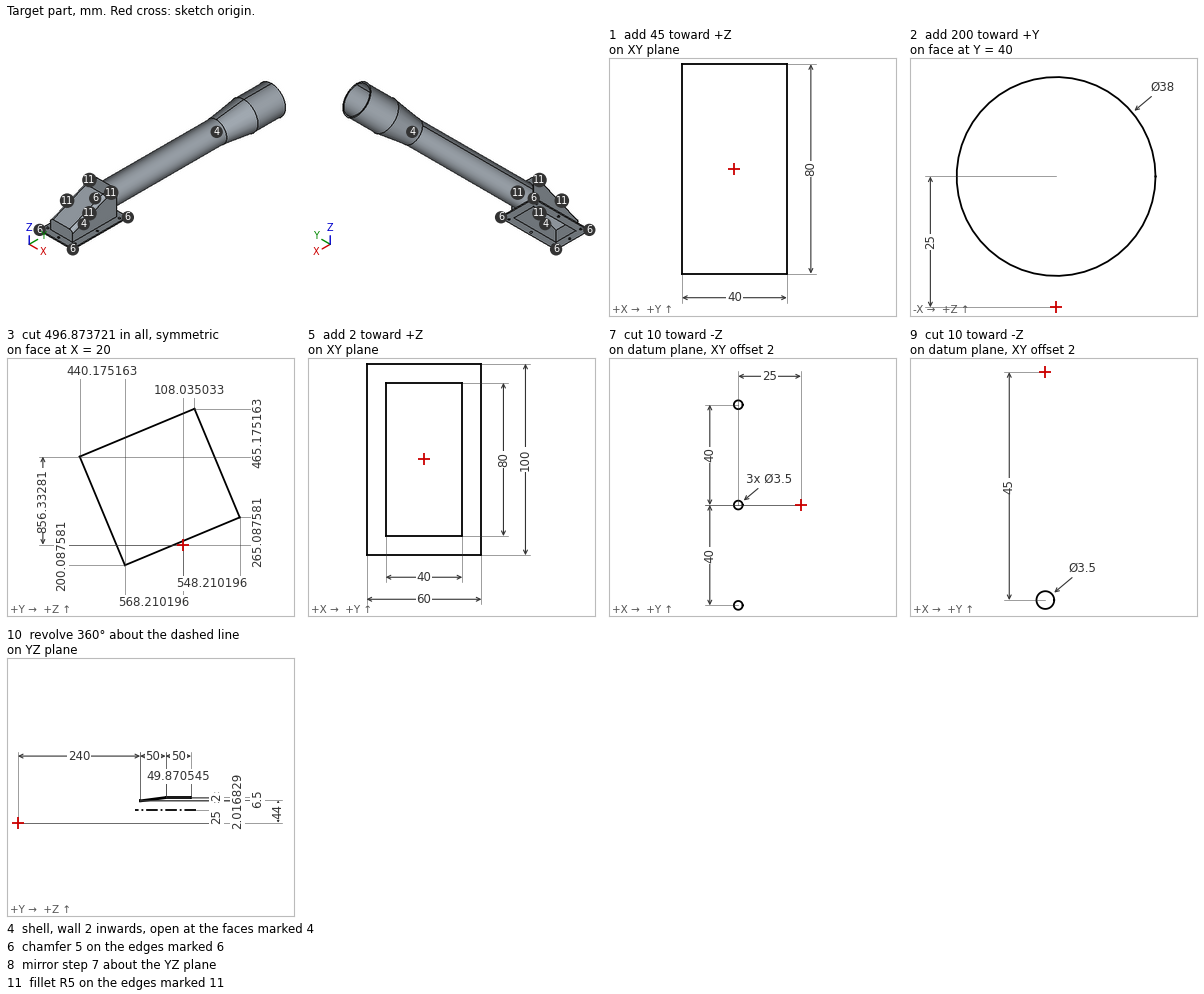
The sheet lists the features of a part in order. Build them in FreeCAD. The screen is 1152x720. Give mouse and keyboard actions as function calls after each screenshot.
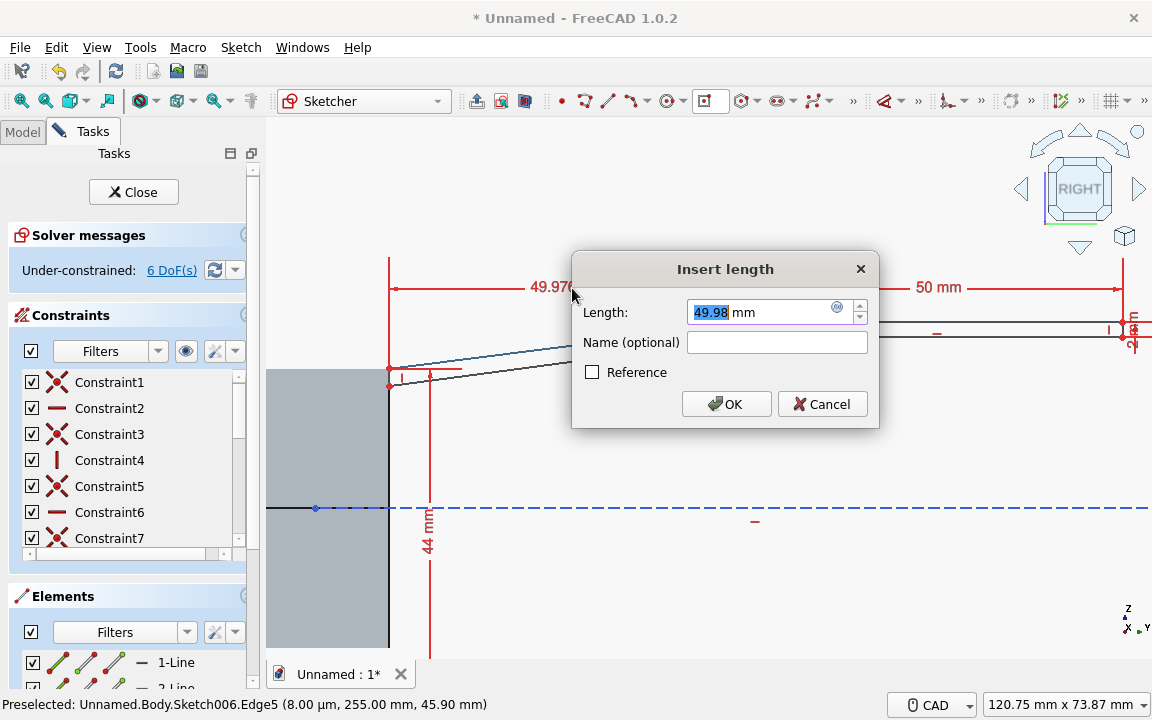
text(50)
key(Return)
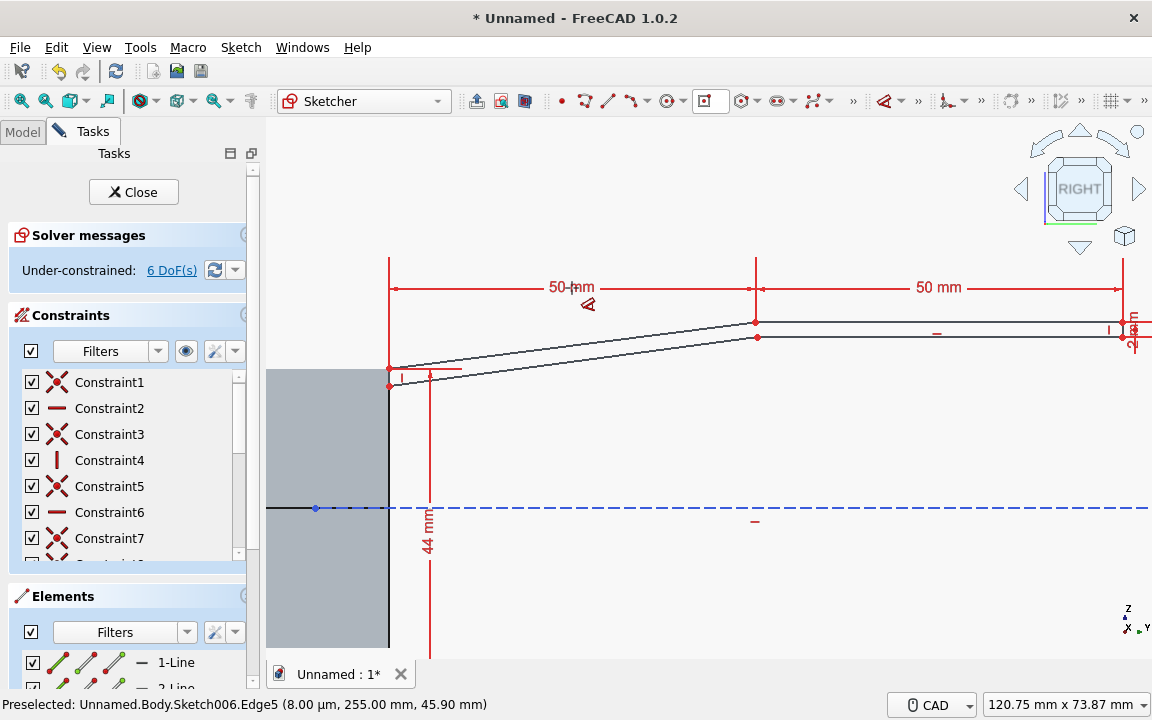
click(389, 386)
click(342, 352)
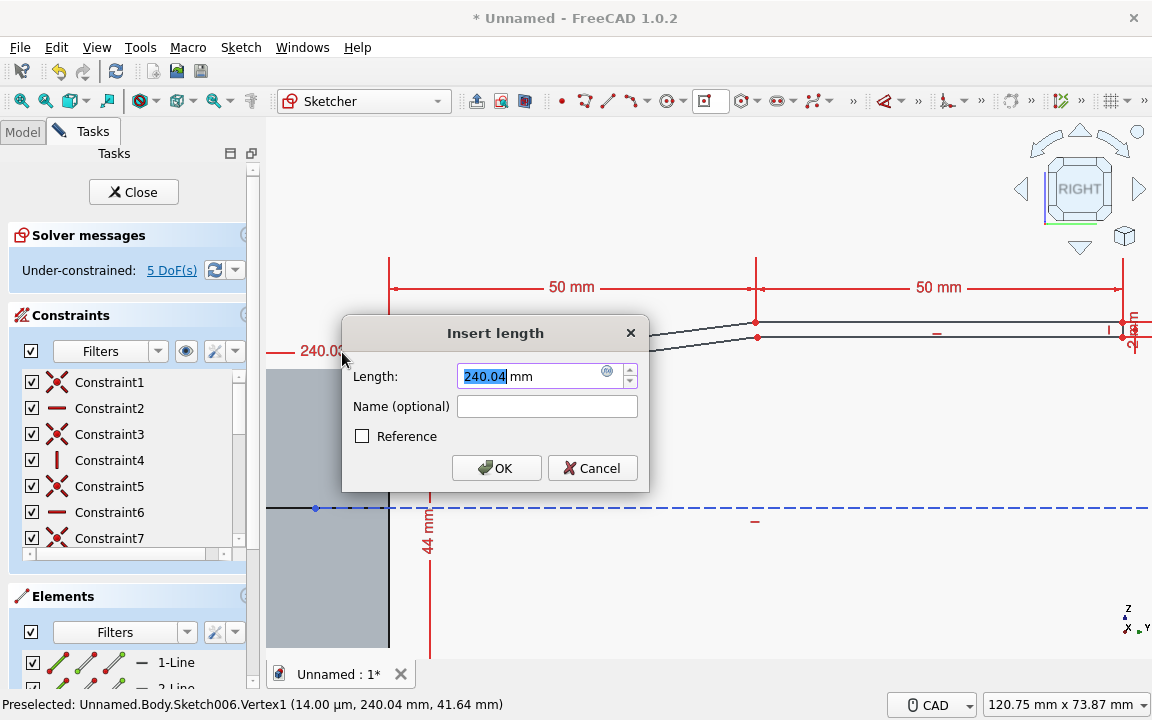
text(240)
key(Return)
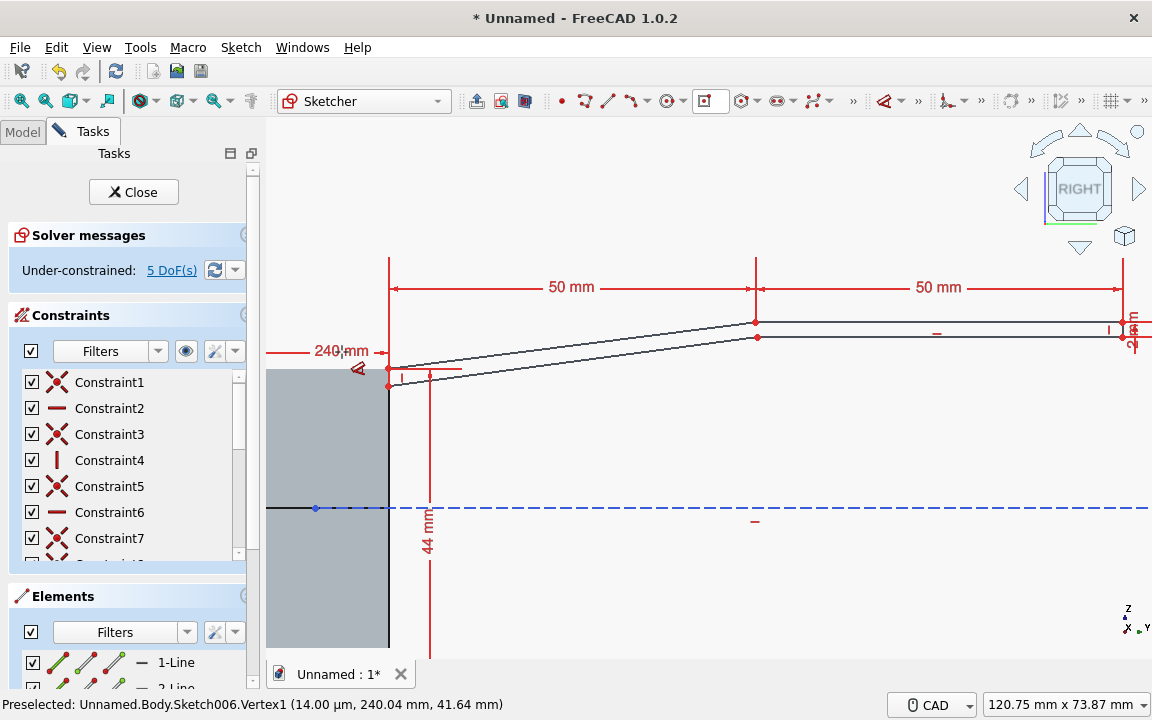
click(646, 336)
click(355, 329)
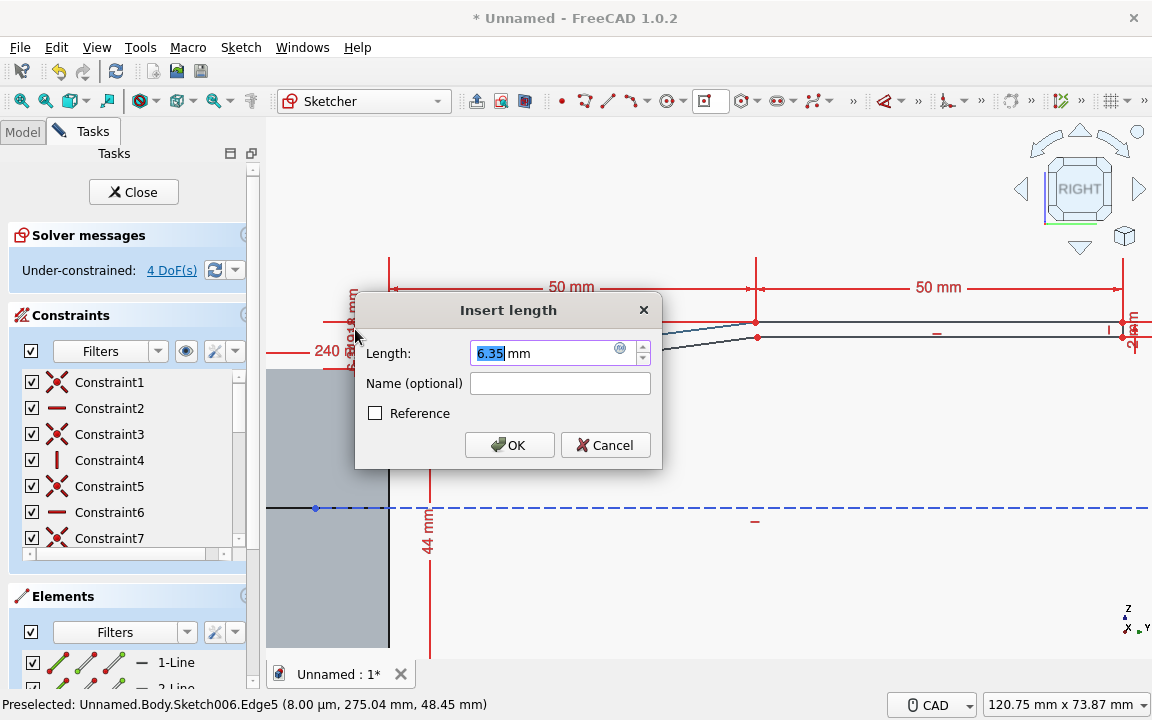
text(6.5)
key(Return)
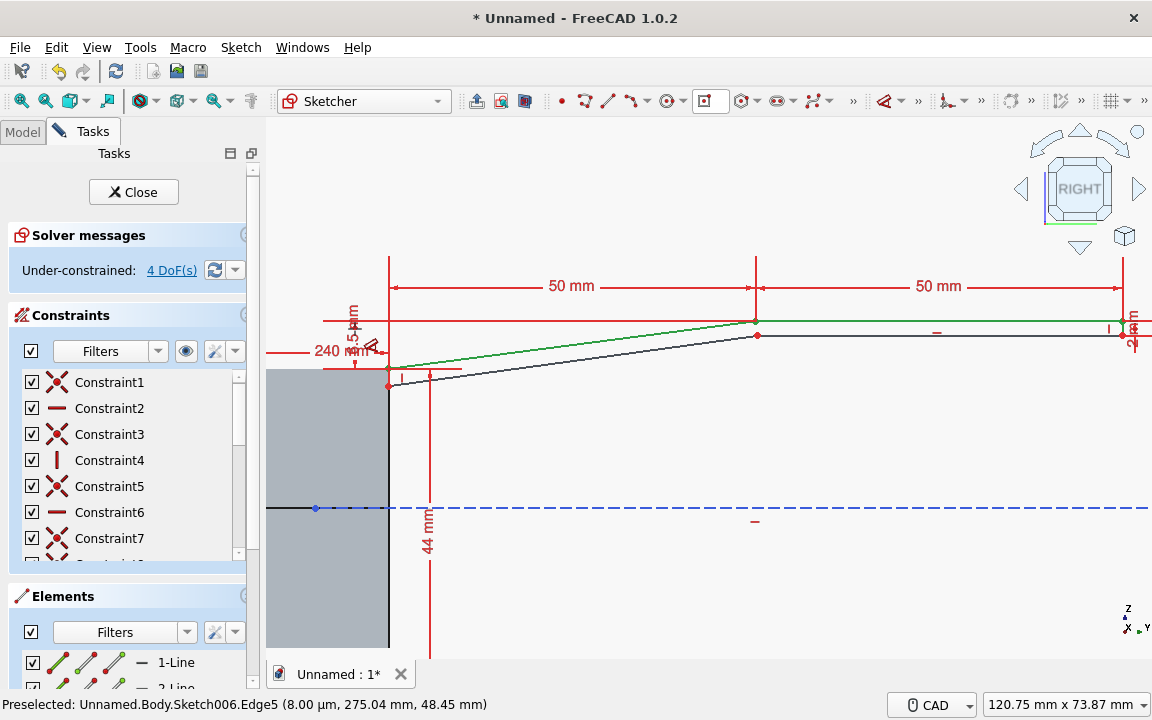
scroll(389, 378, up, 5)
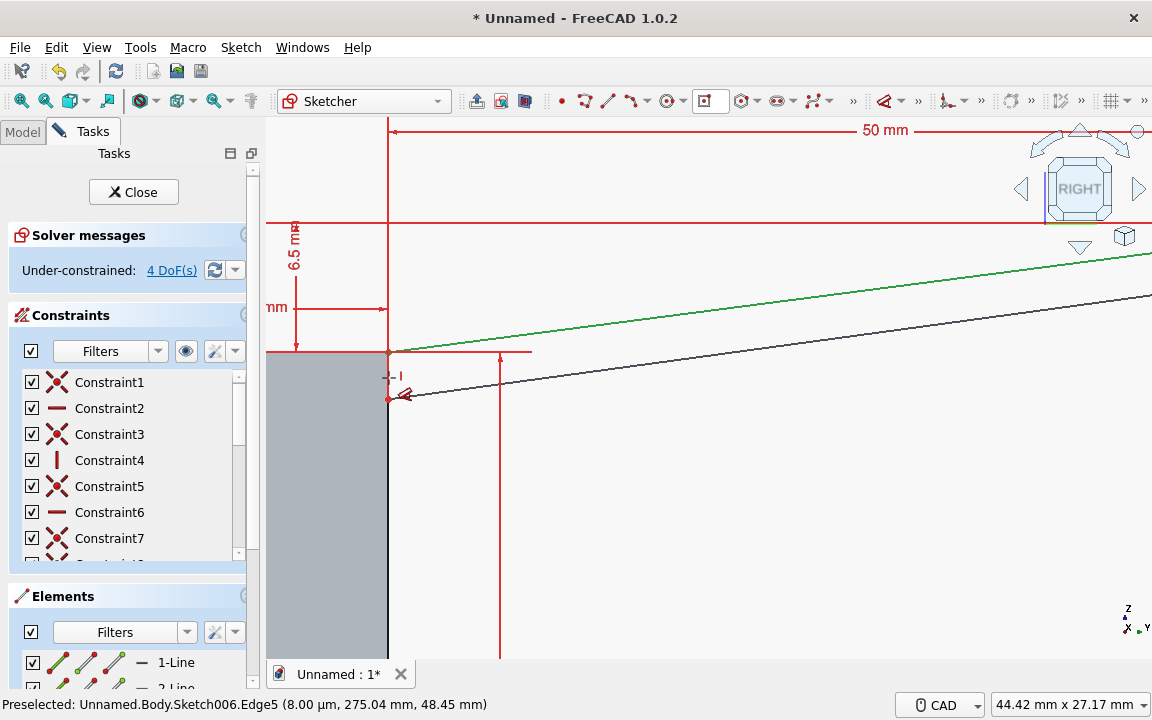
click(388, 376)
click(354, 376)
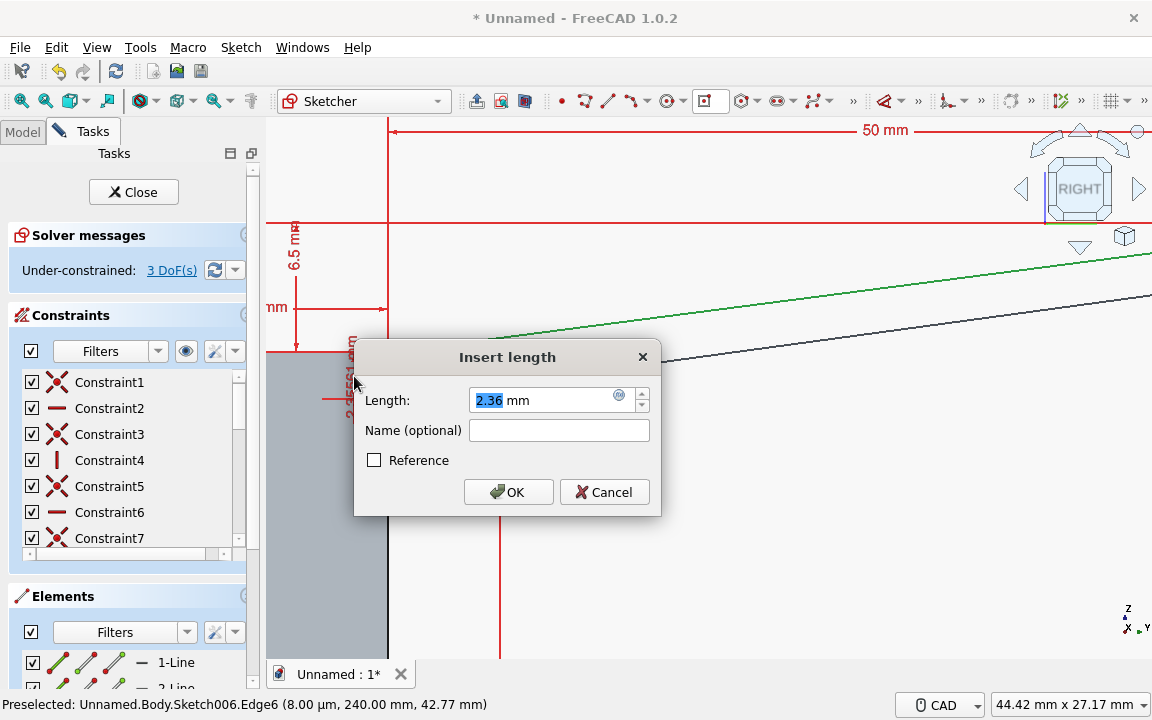
text(2.016829)
key(Return)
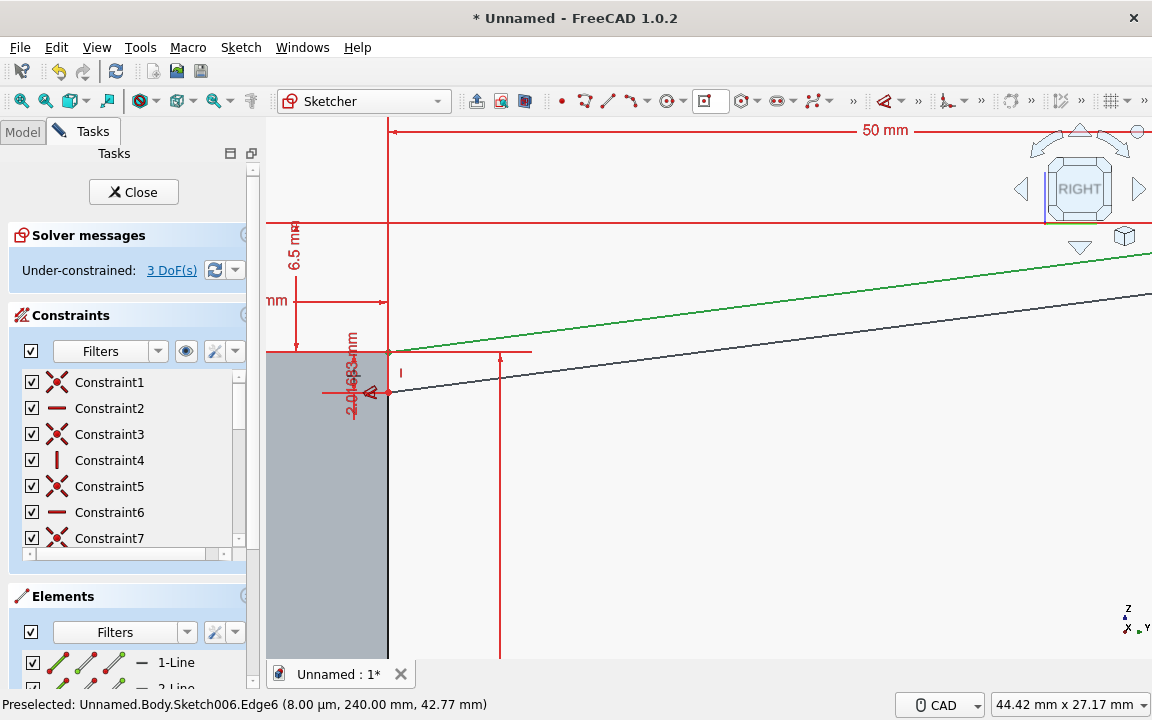
scroll(452, 365, down, 8)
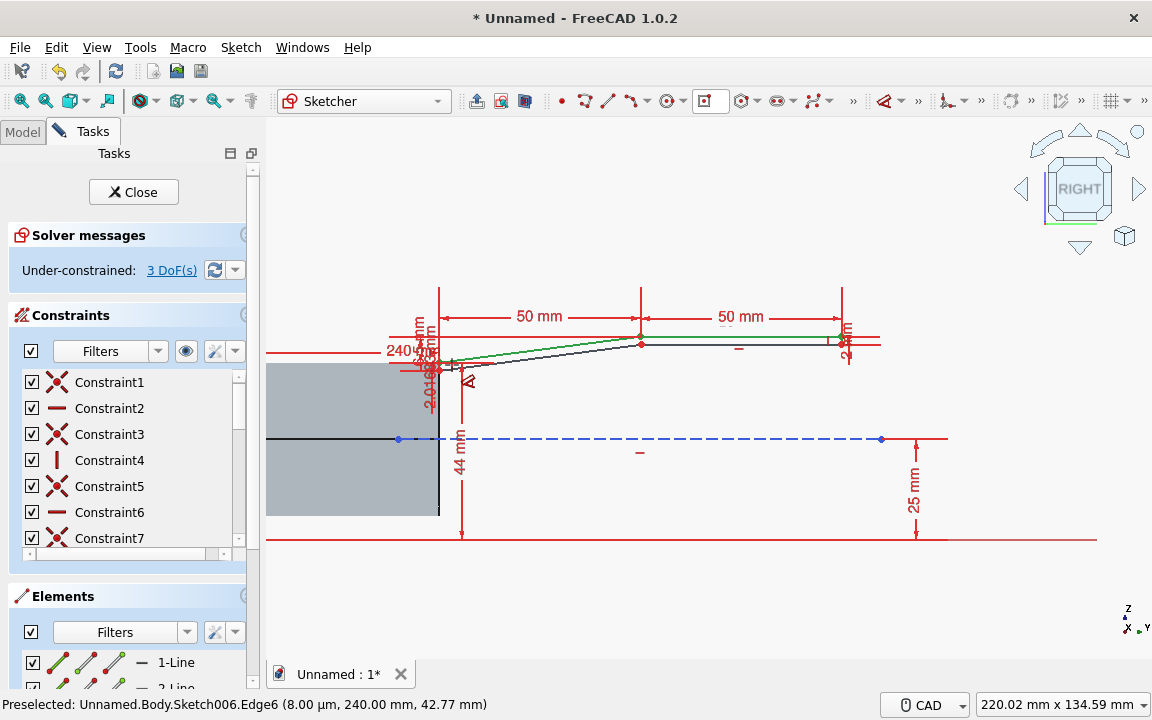
scroll(702, 345, up, 3)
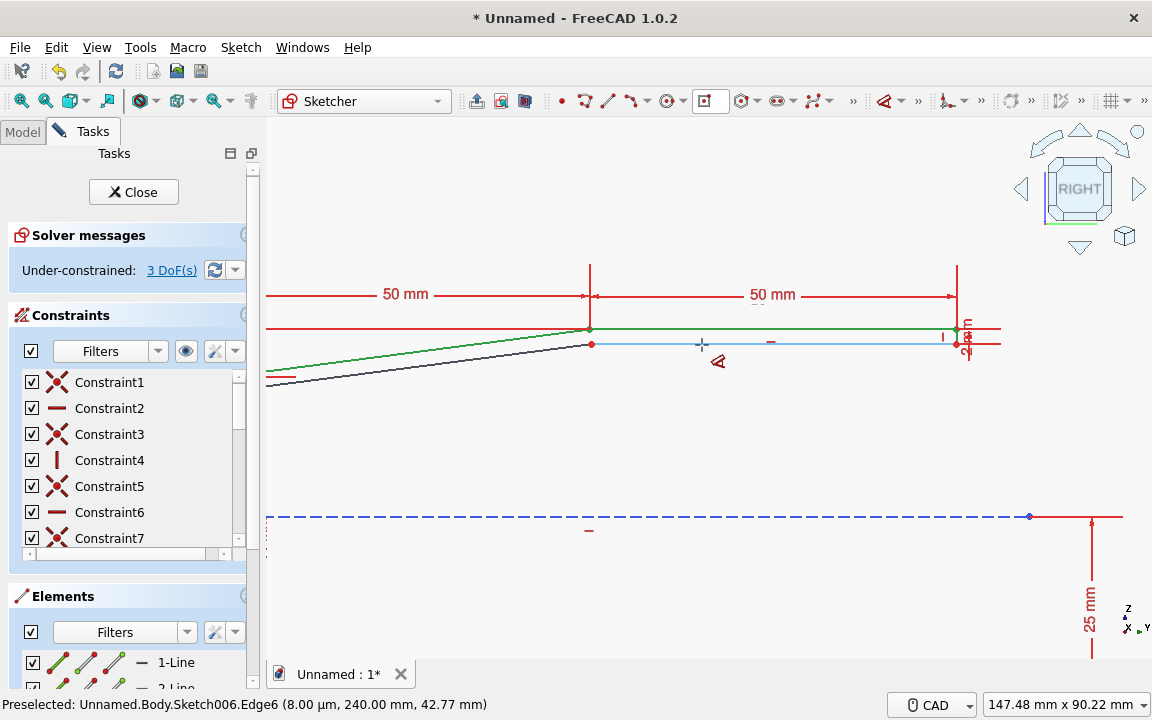
click(701, 344)
click(690, 310)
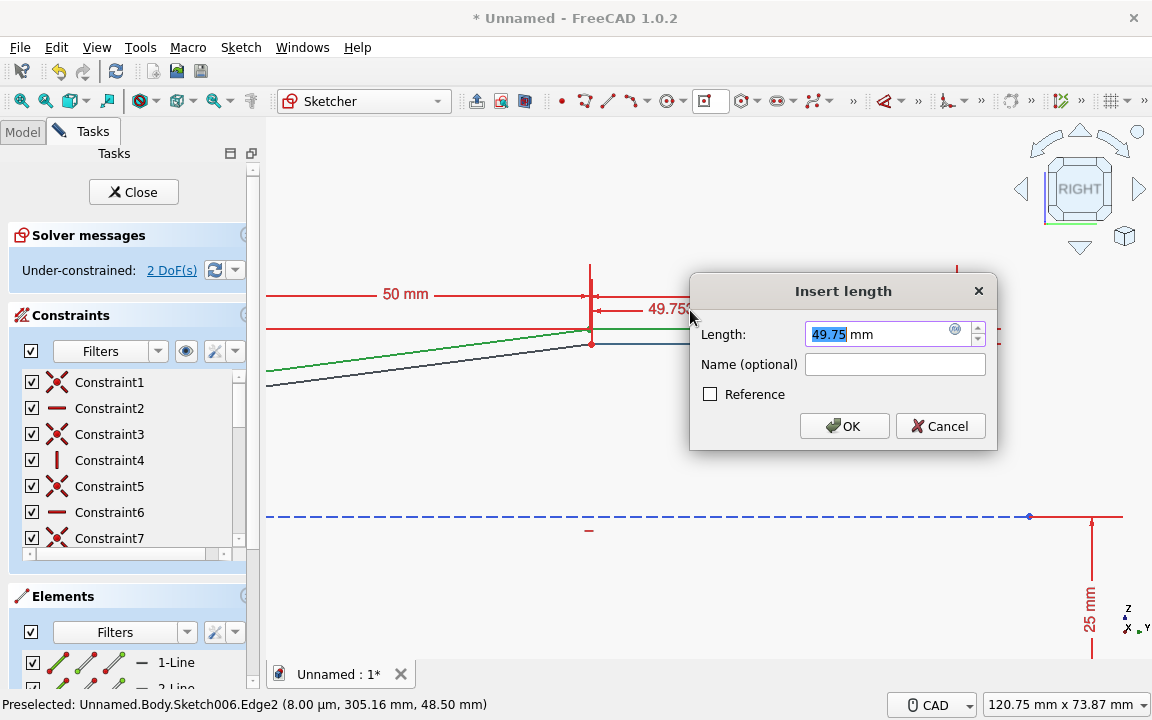
text(49.870545)
key(Return)
key(Escape)